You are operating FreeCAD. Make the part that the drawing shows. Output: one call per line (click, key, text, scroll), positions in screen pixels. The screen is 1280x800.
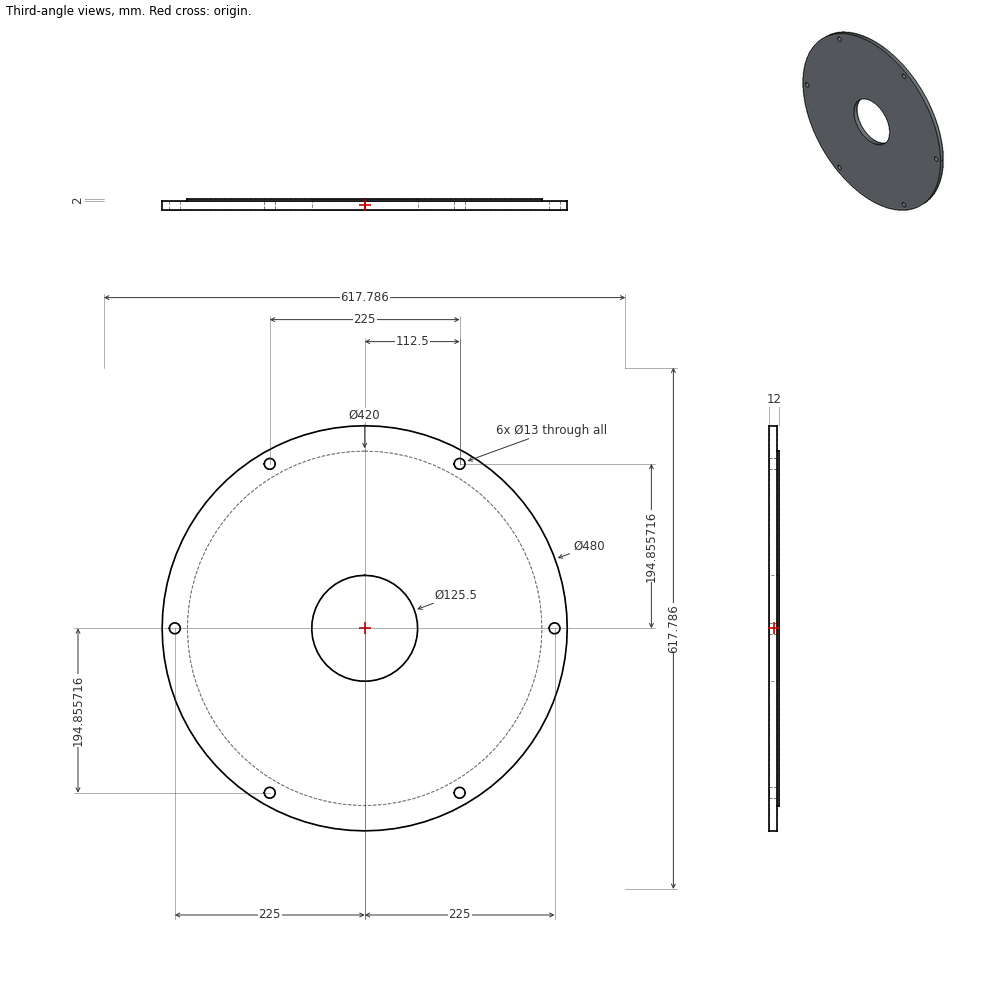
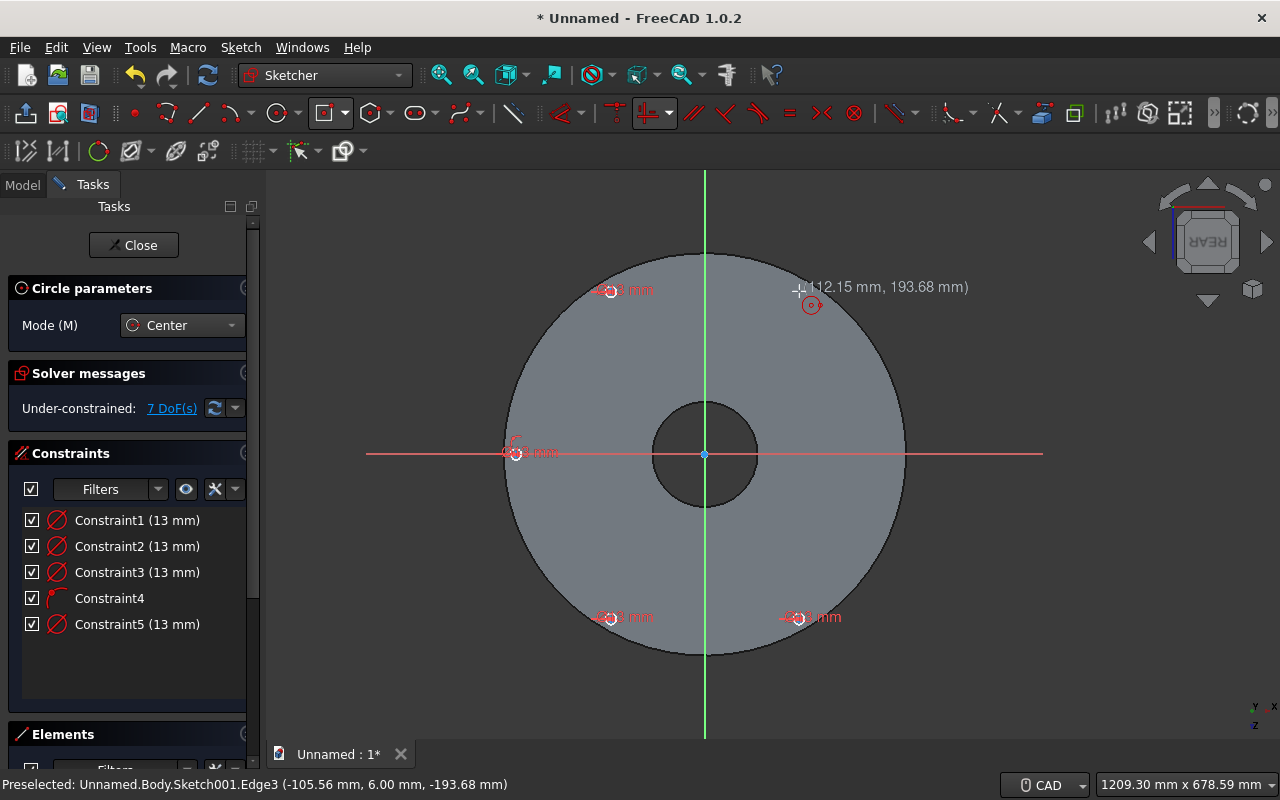
click(799, 291)
move(803, 287)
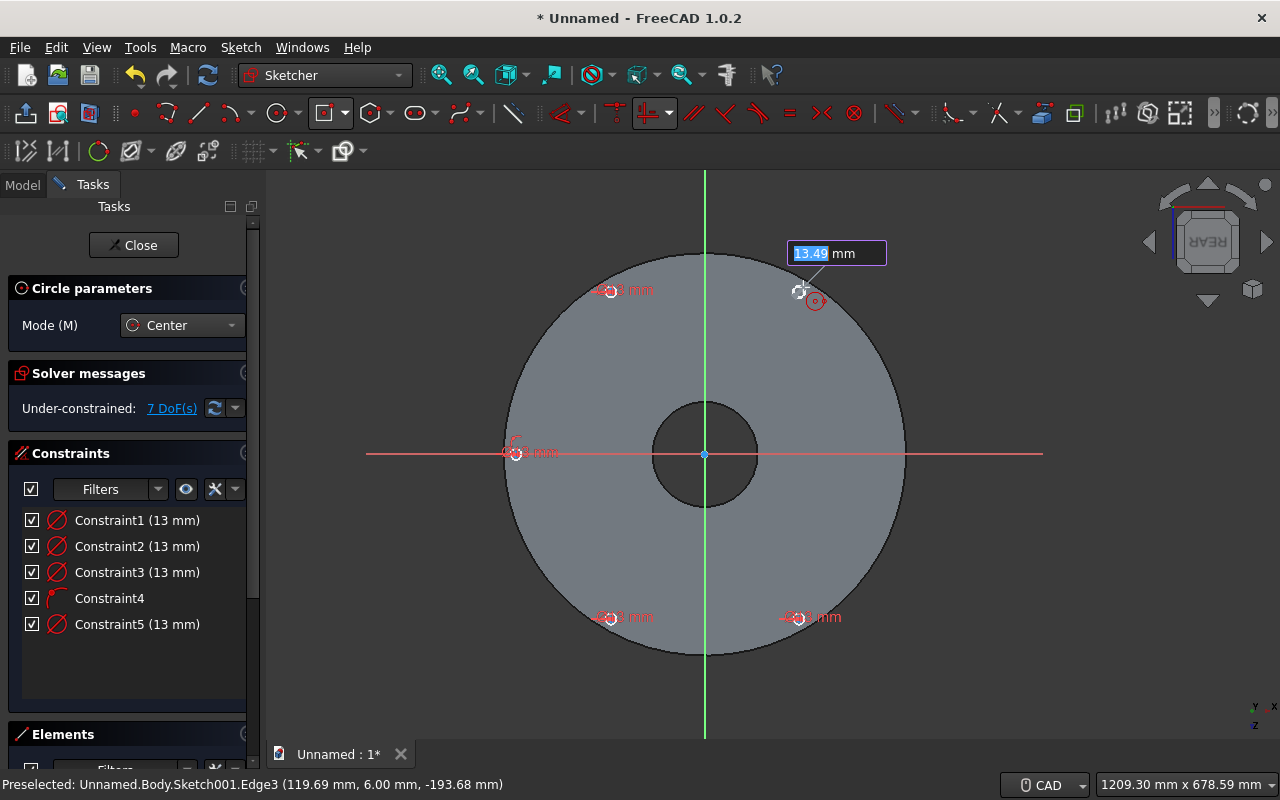
text(13)
key(Return)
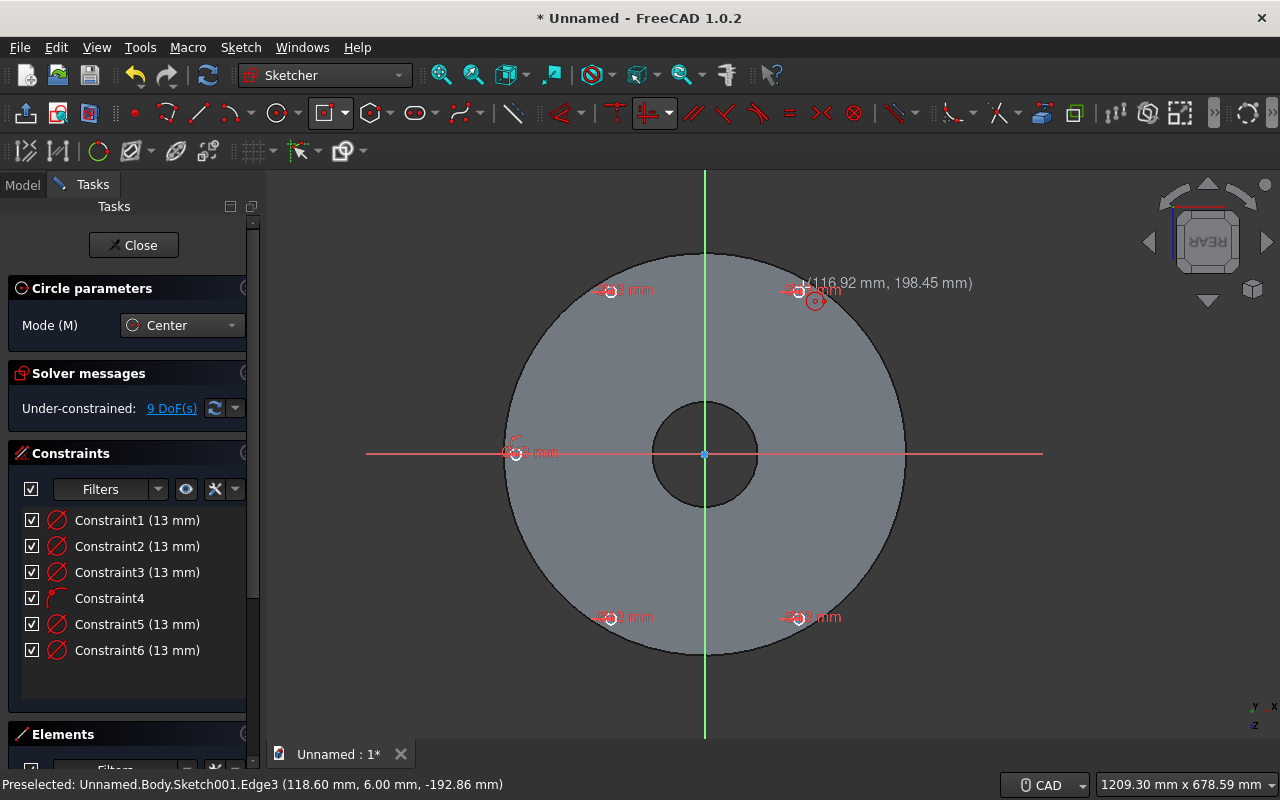
scroll(894, 454, up, 8)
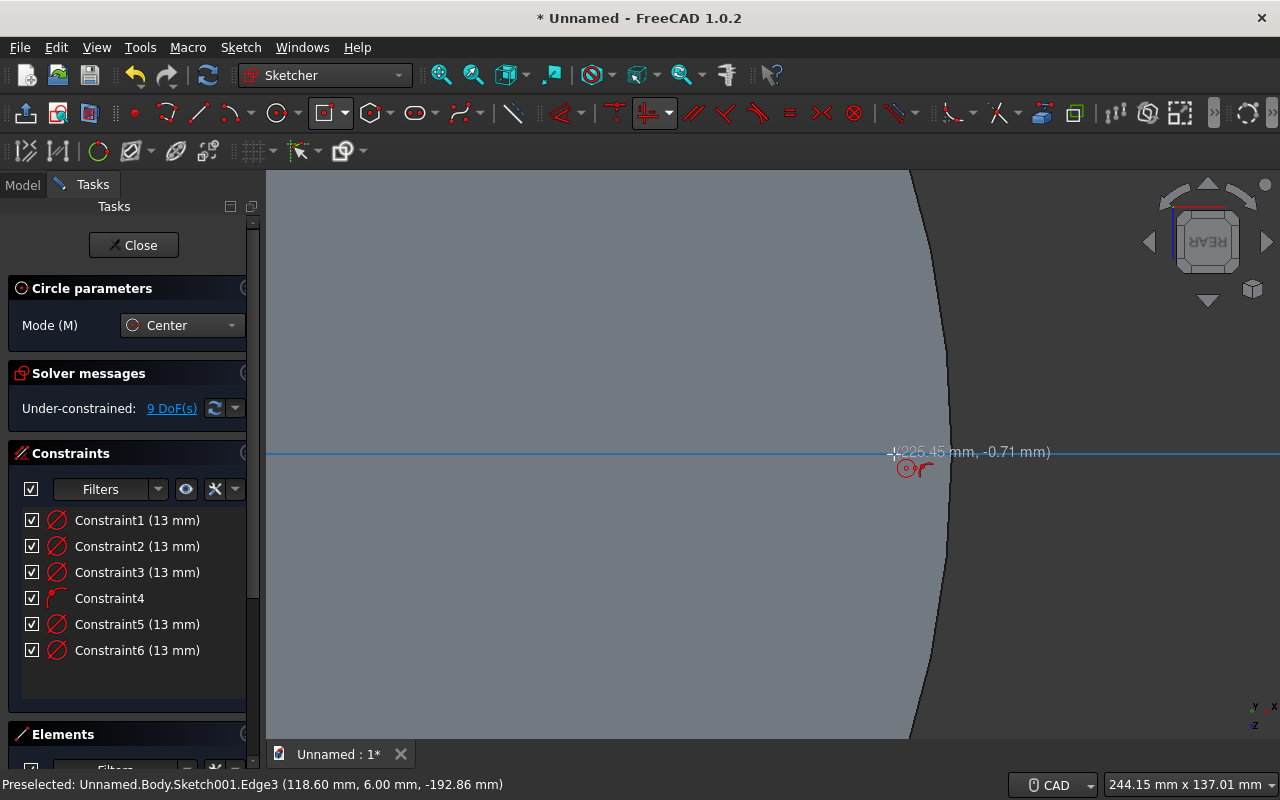
scroll(894, 455, down, 8)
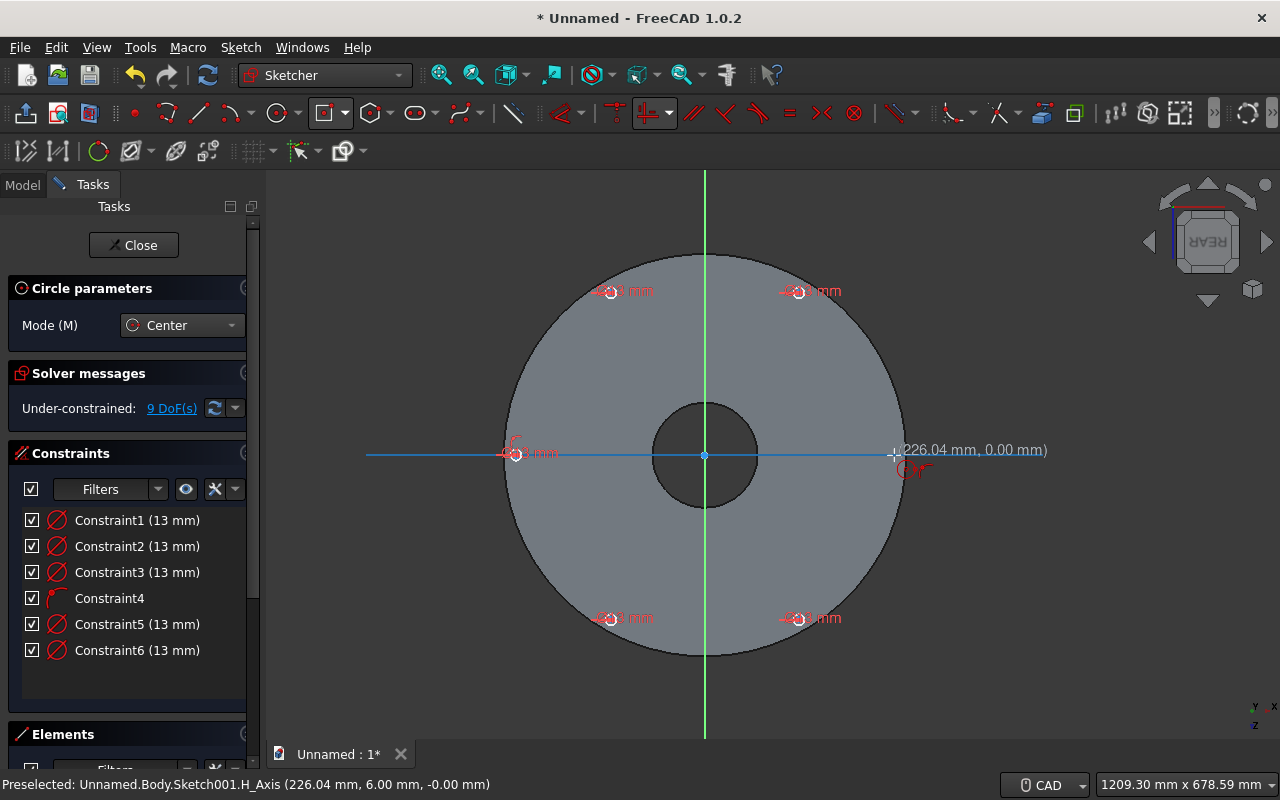
click(894, 455)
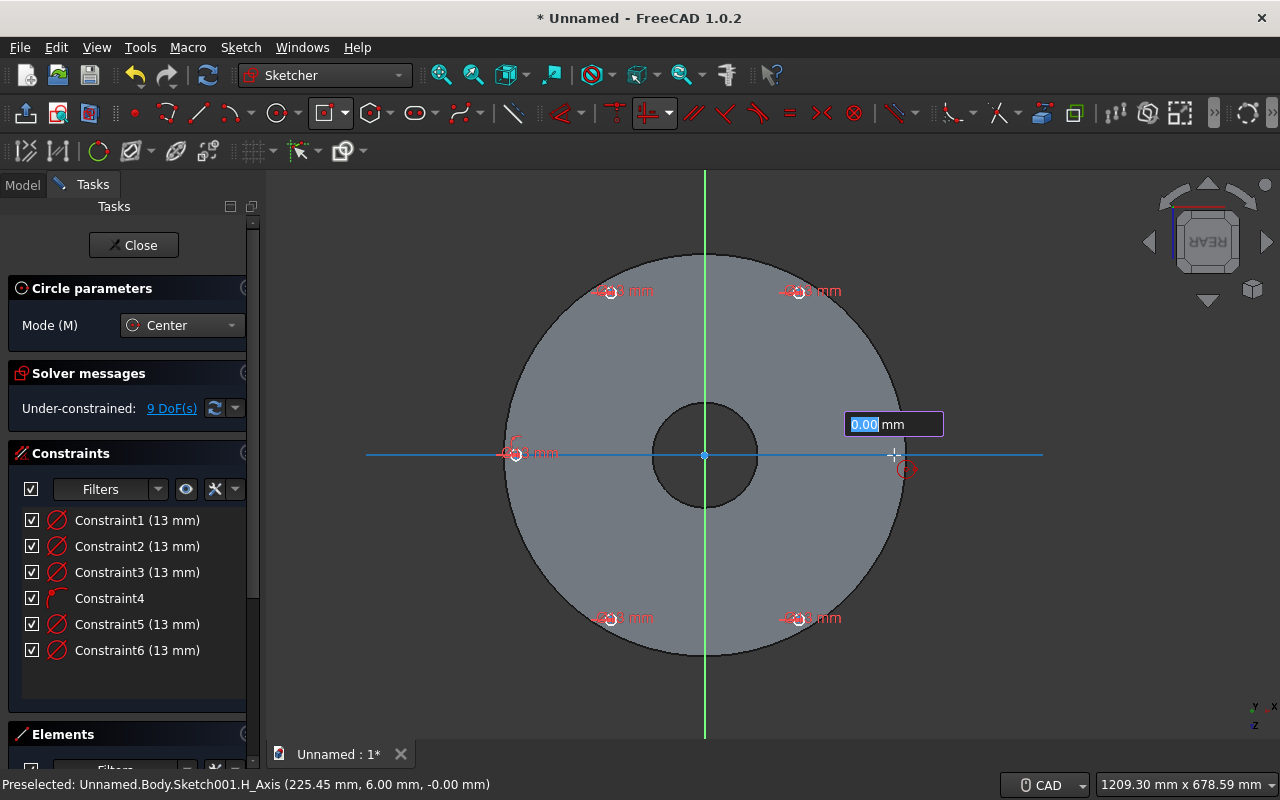
scroll(892, 460, up, 6)
move(890, 460)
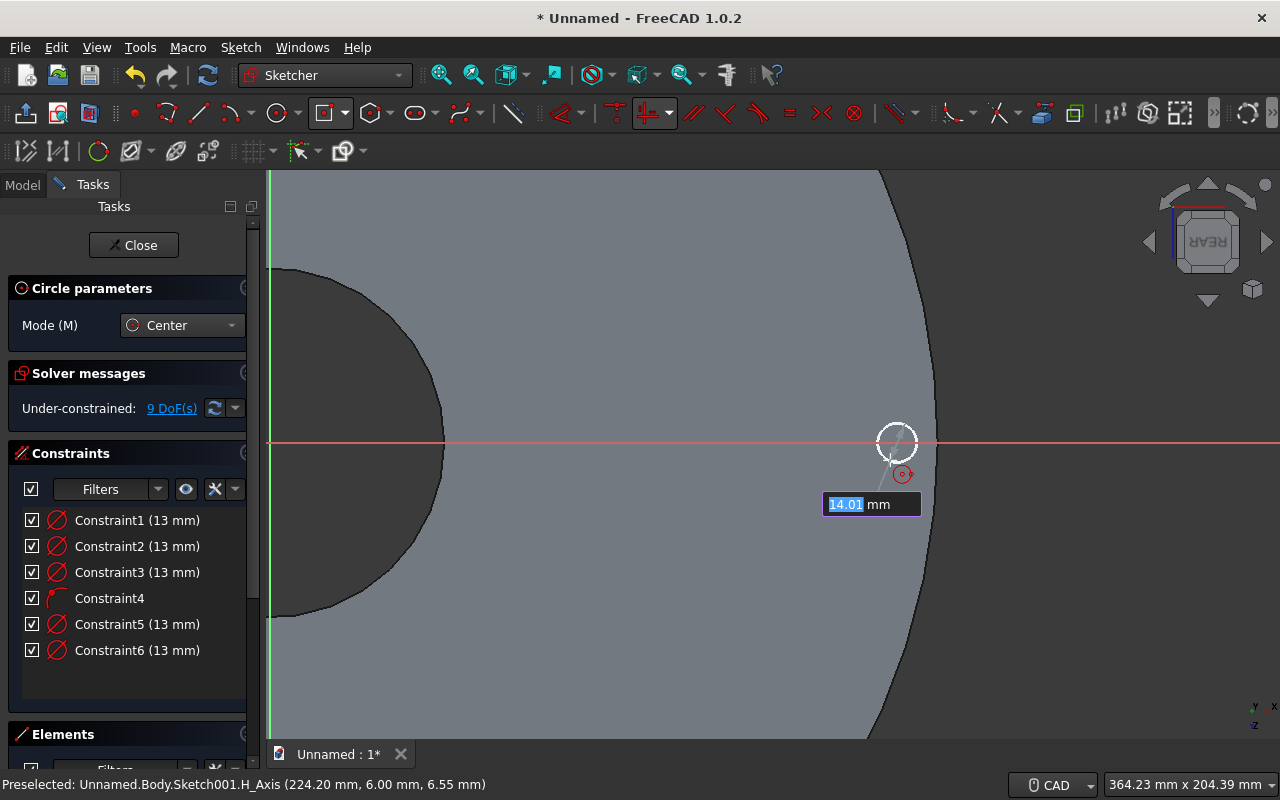
text(13)
key(Return)
key(Escape)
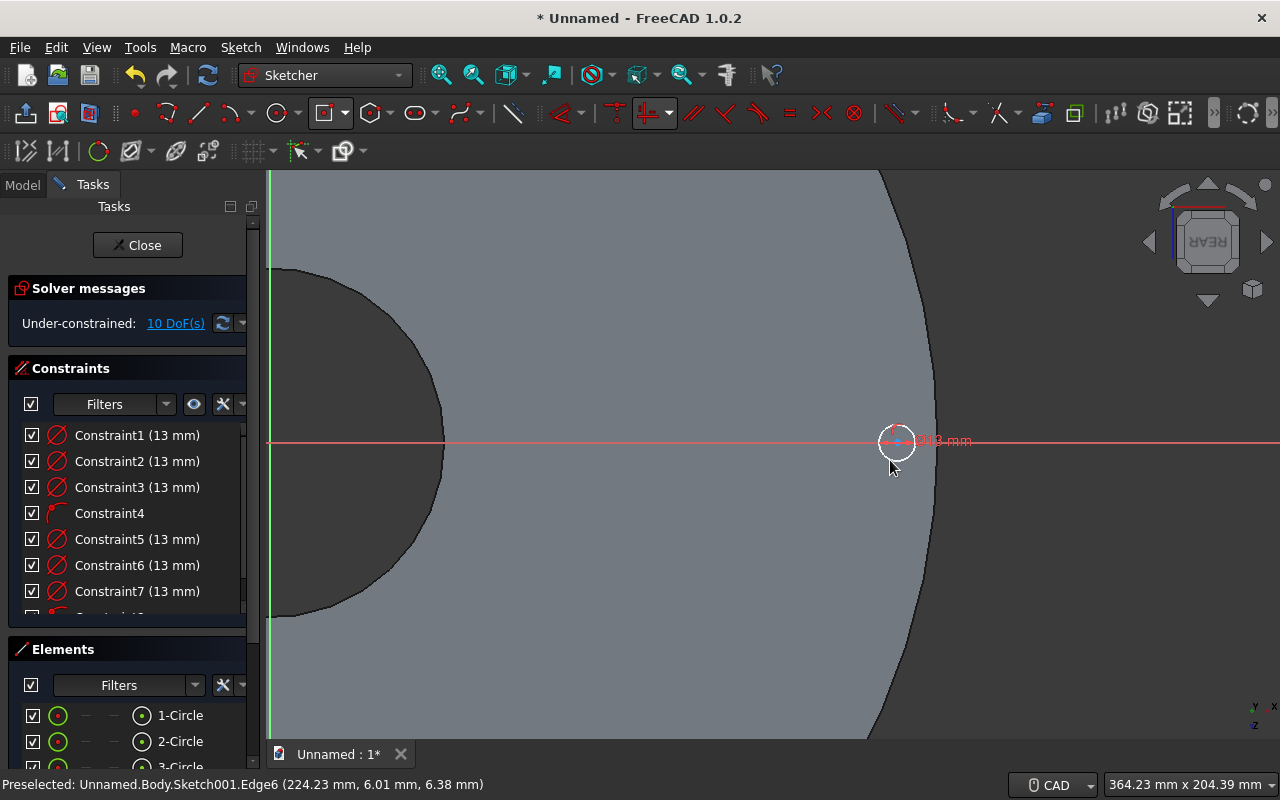
scroll(892, 460, down, 6)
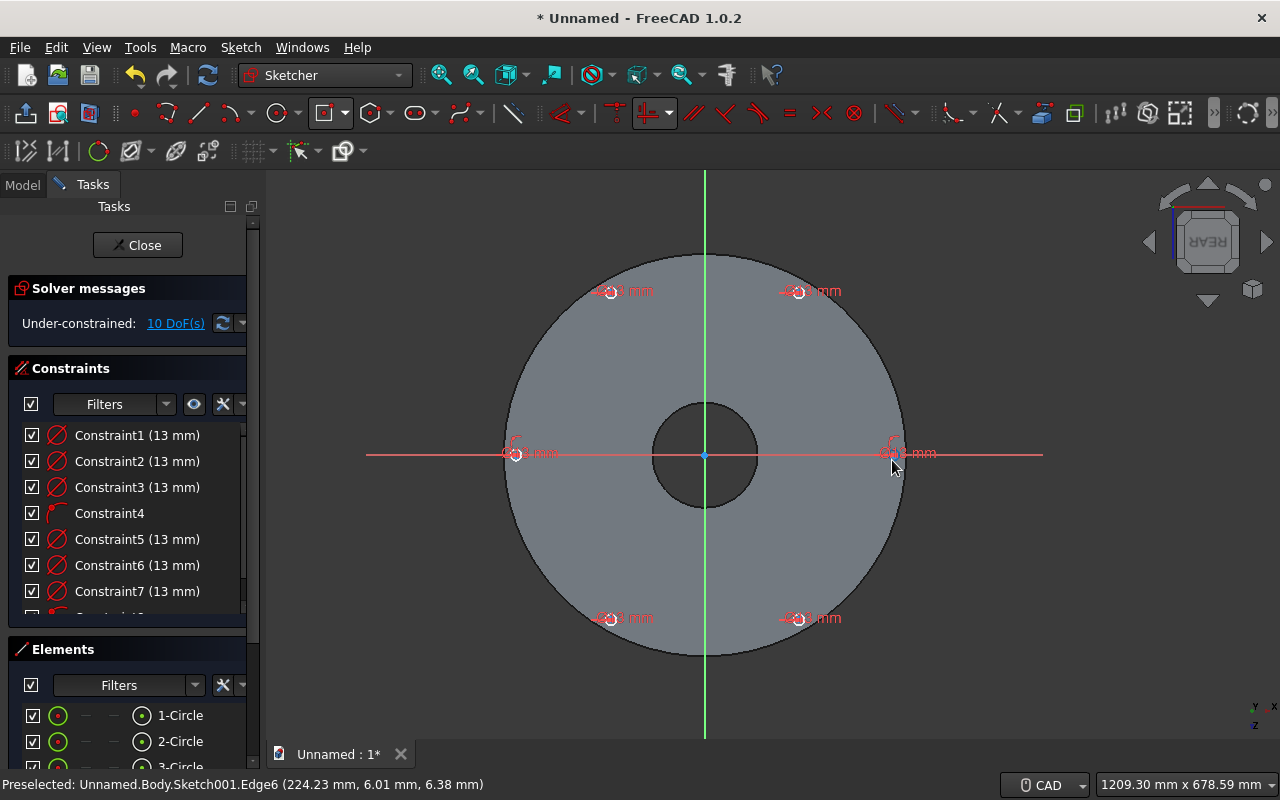
click(799, 620)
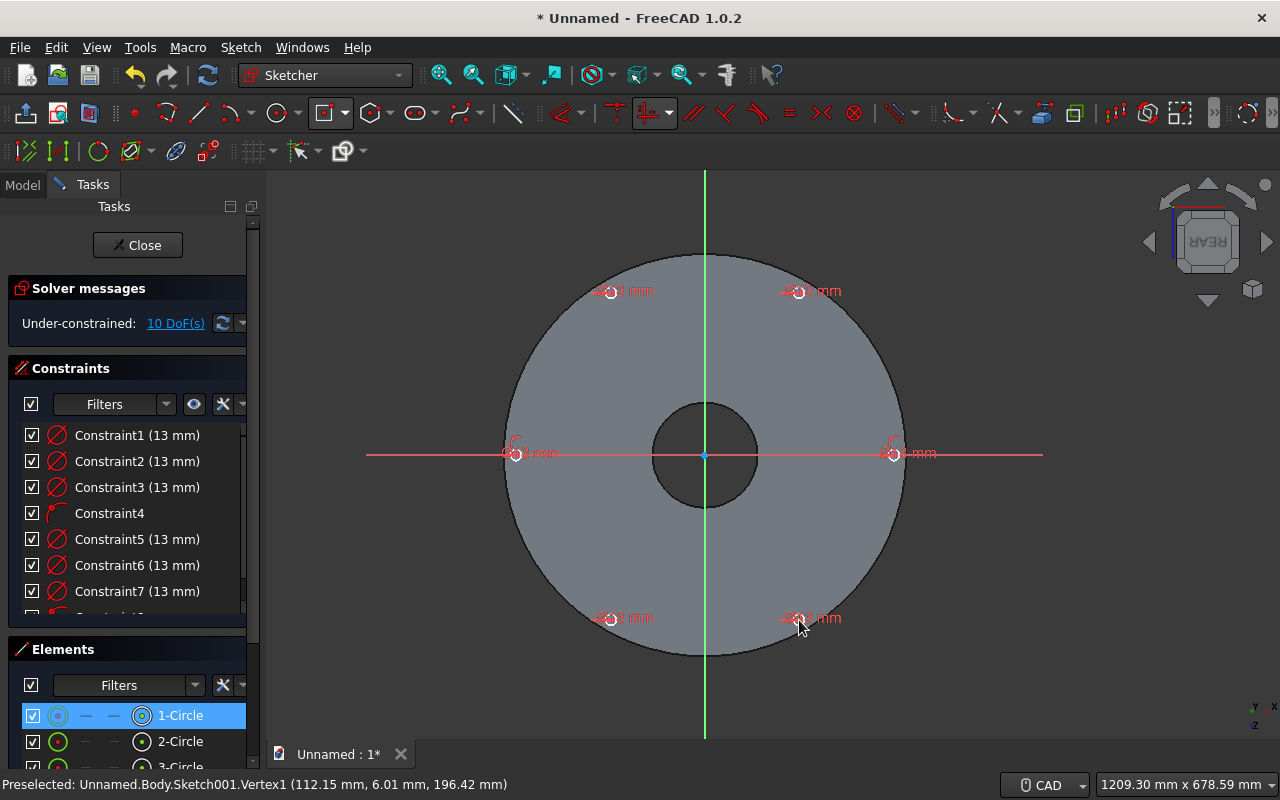
click(611, 620)